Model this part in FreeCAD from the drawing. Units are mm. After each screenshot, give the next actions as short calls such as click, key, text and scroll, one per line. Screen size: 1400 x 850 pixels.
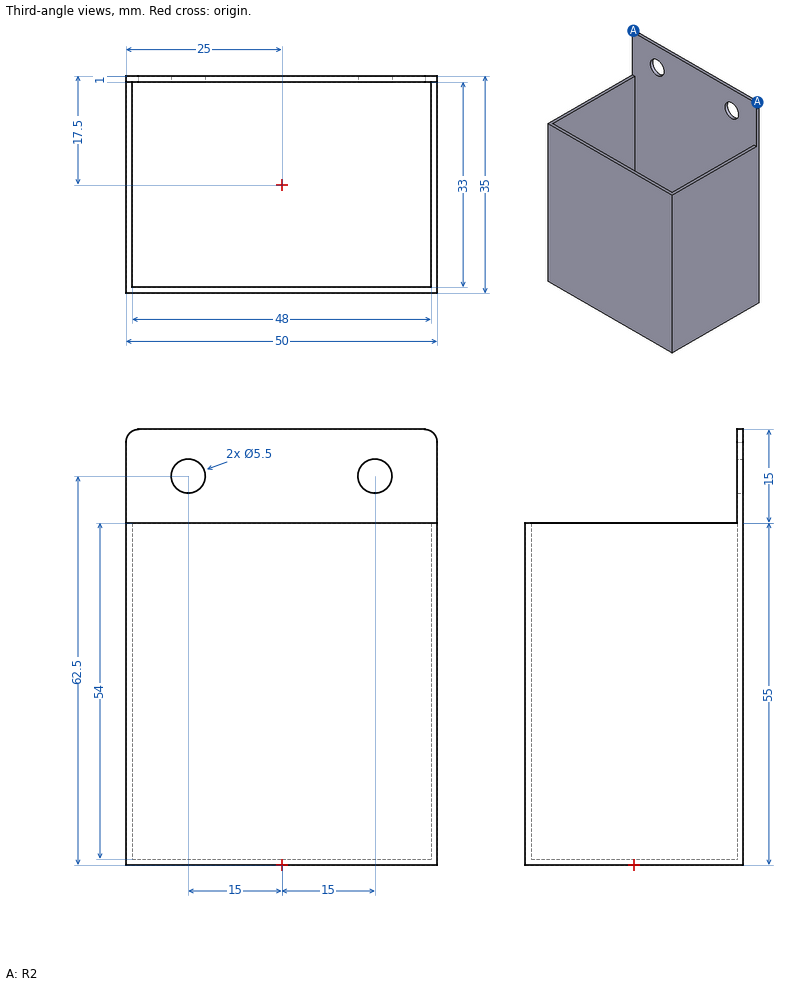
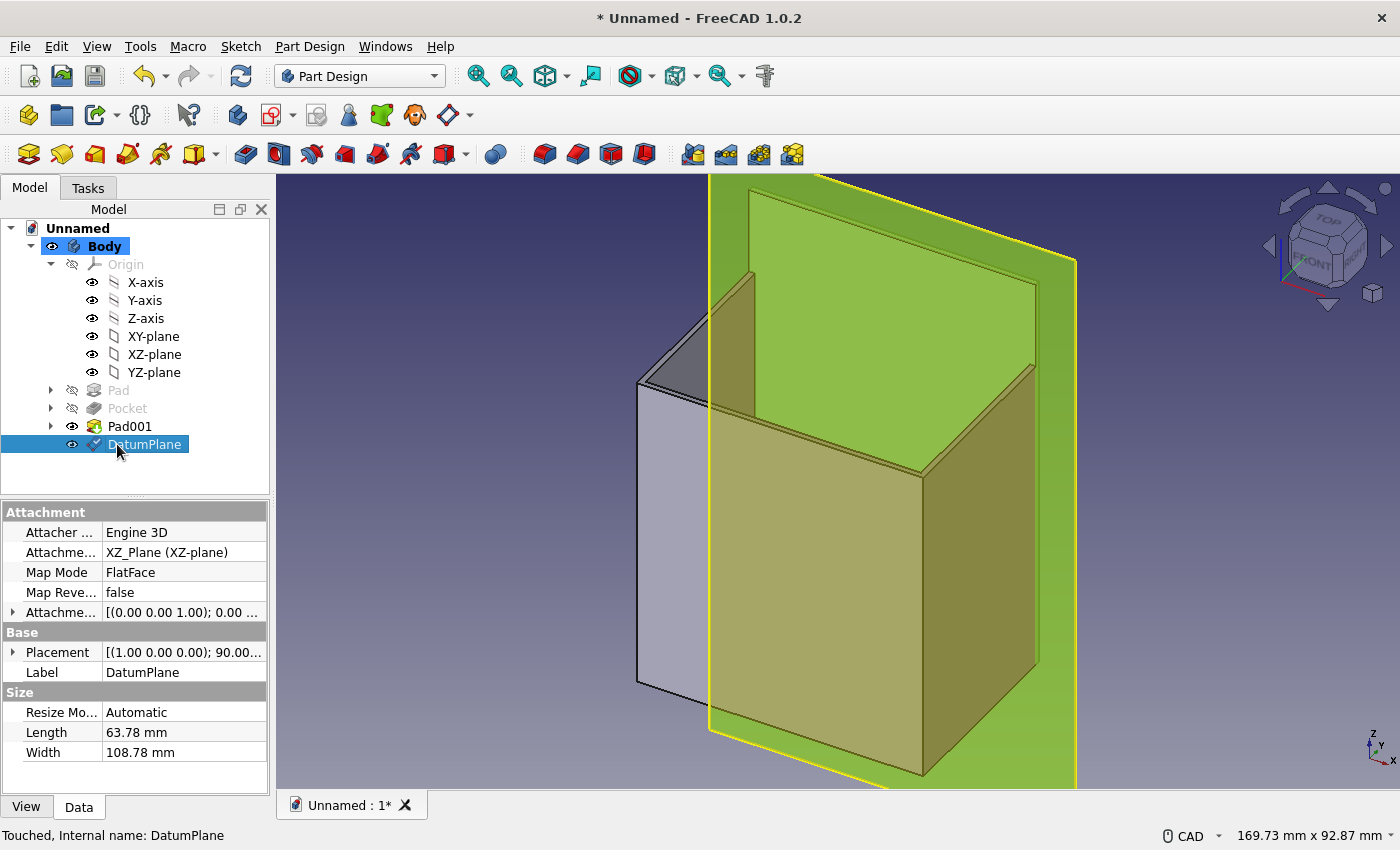
click(270, 116)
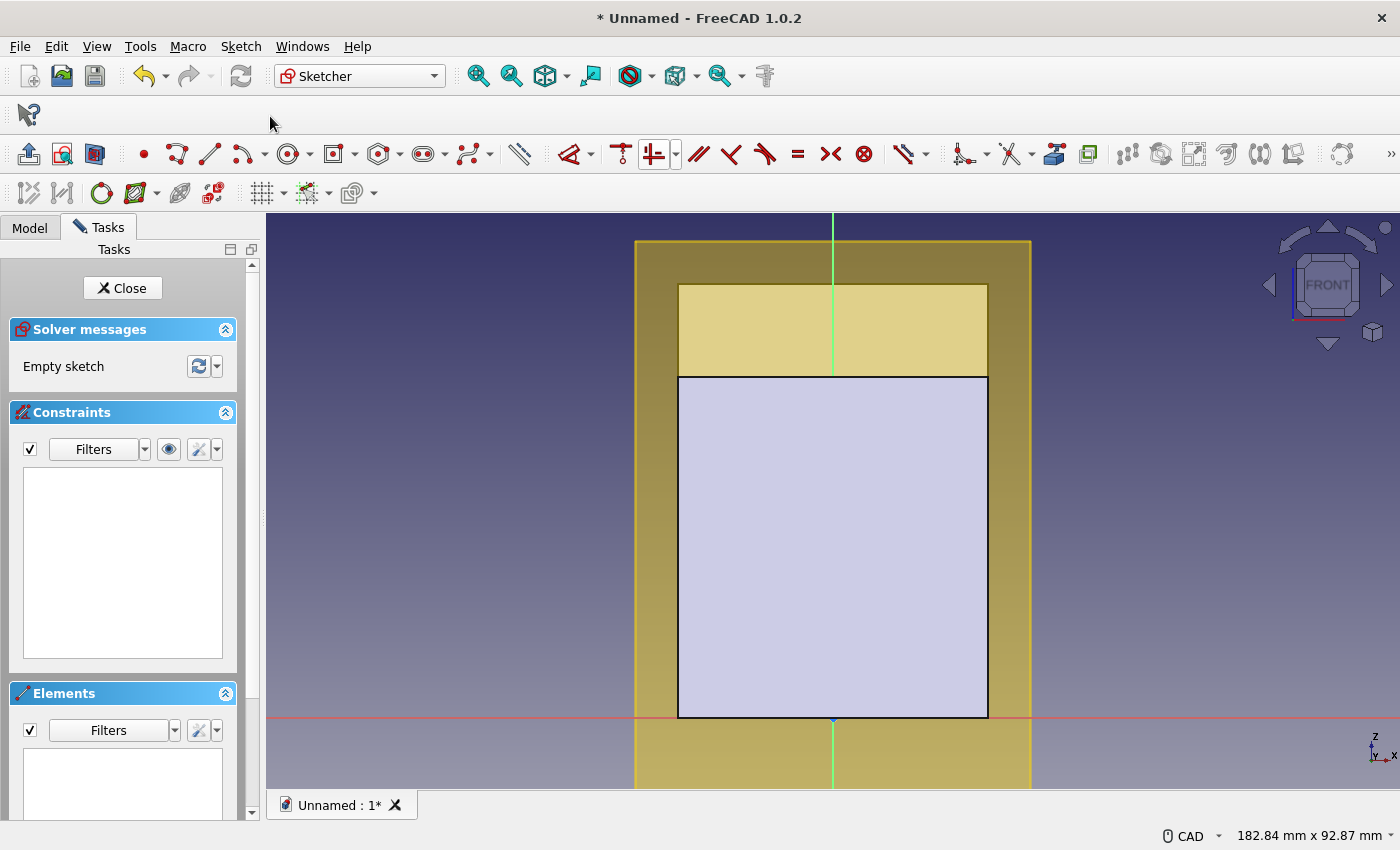
key(q)
key(s)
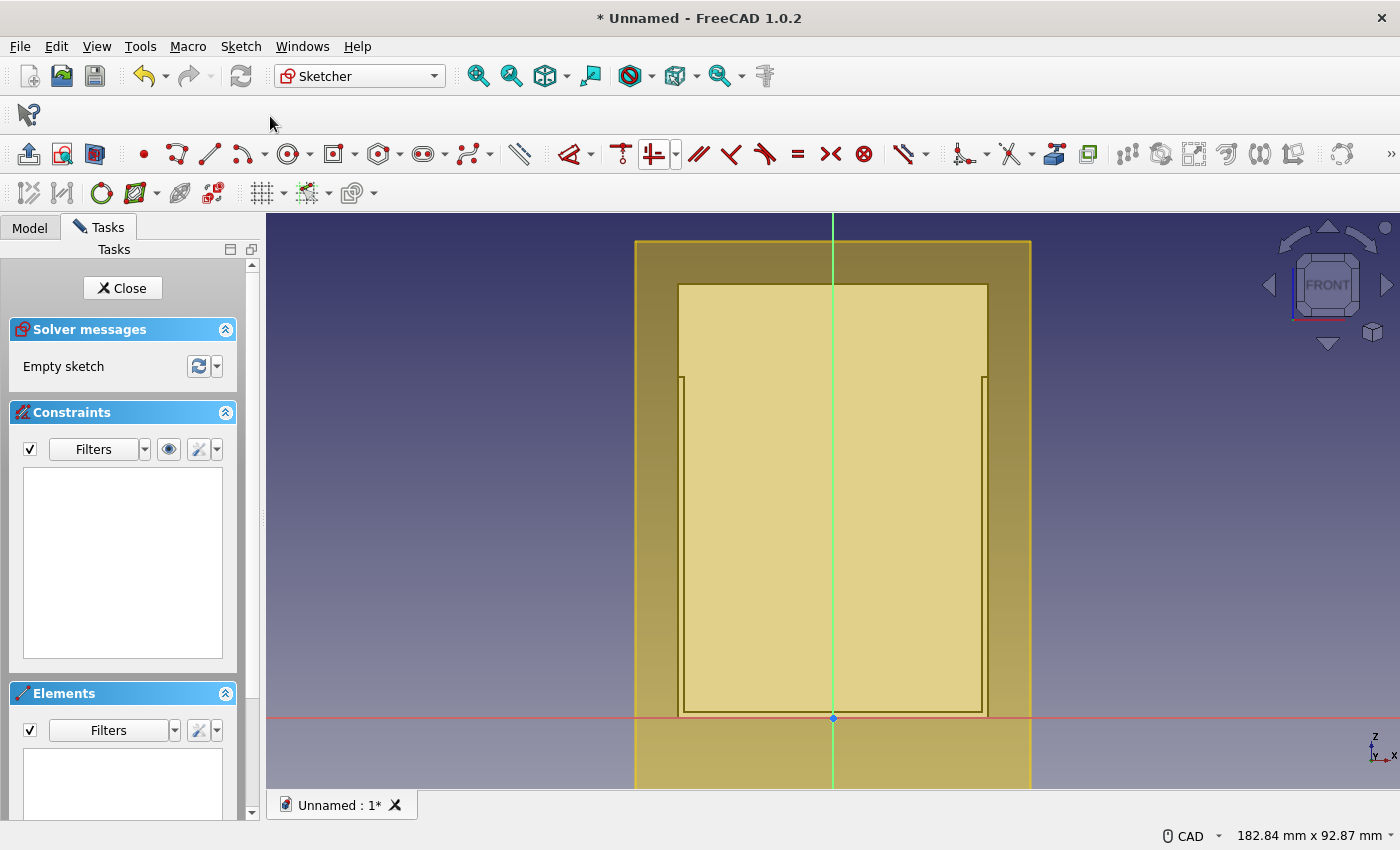
click(288, 154)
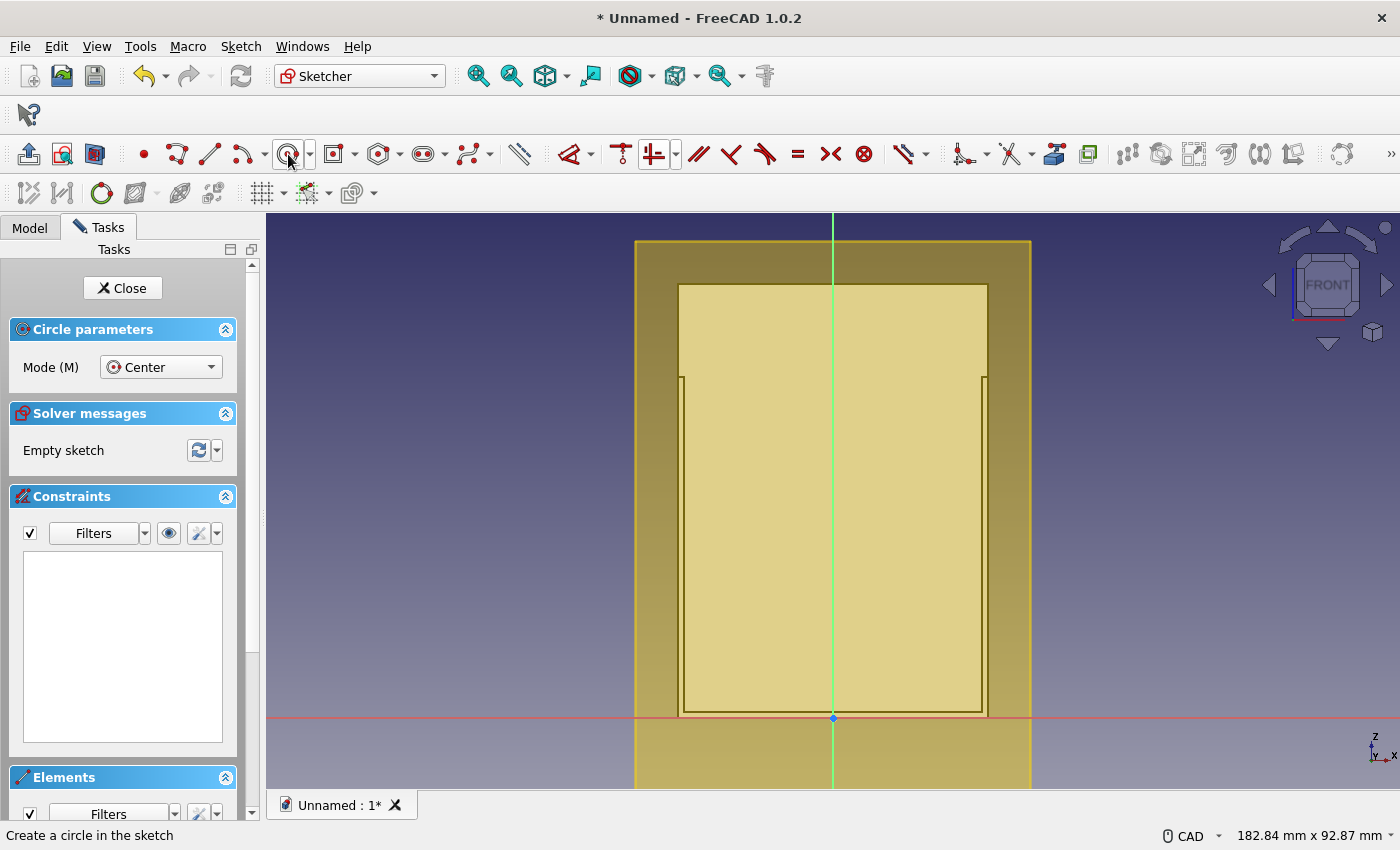
scroll(740, 330, up, 2)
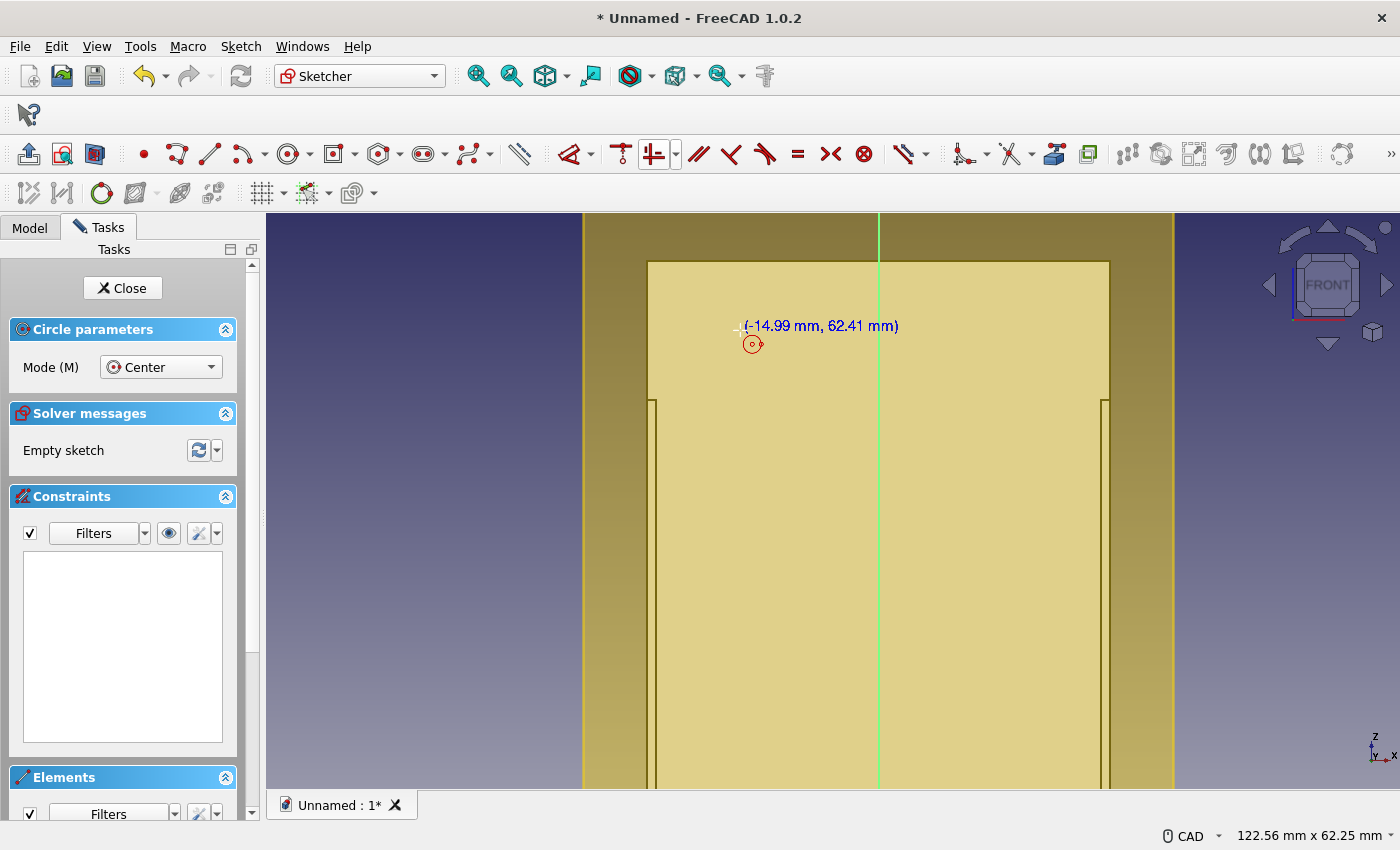
click(740, 331)
click(758, 313)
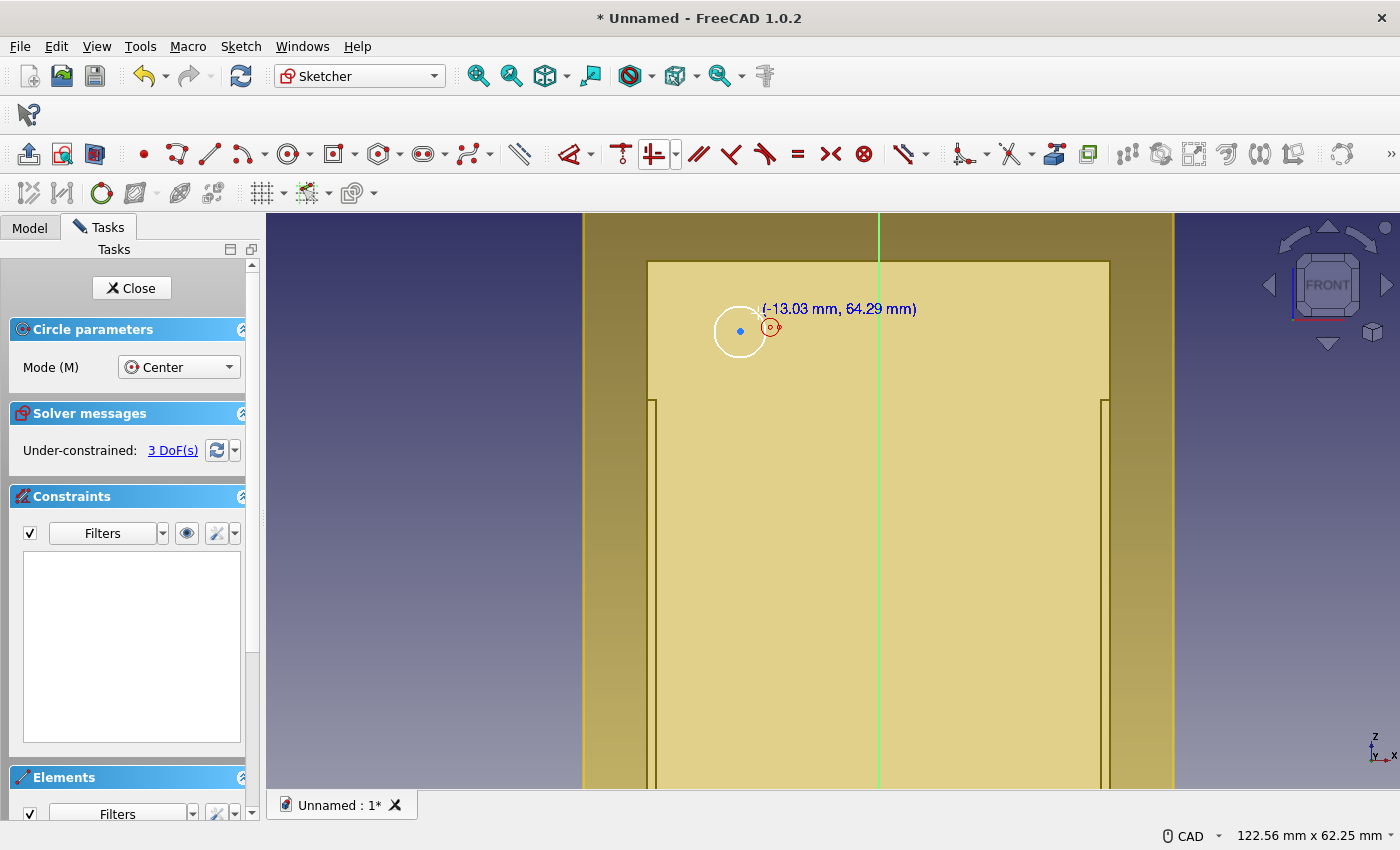
click(1017, 331)
click(1035, 313)
key(Escape)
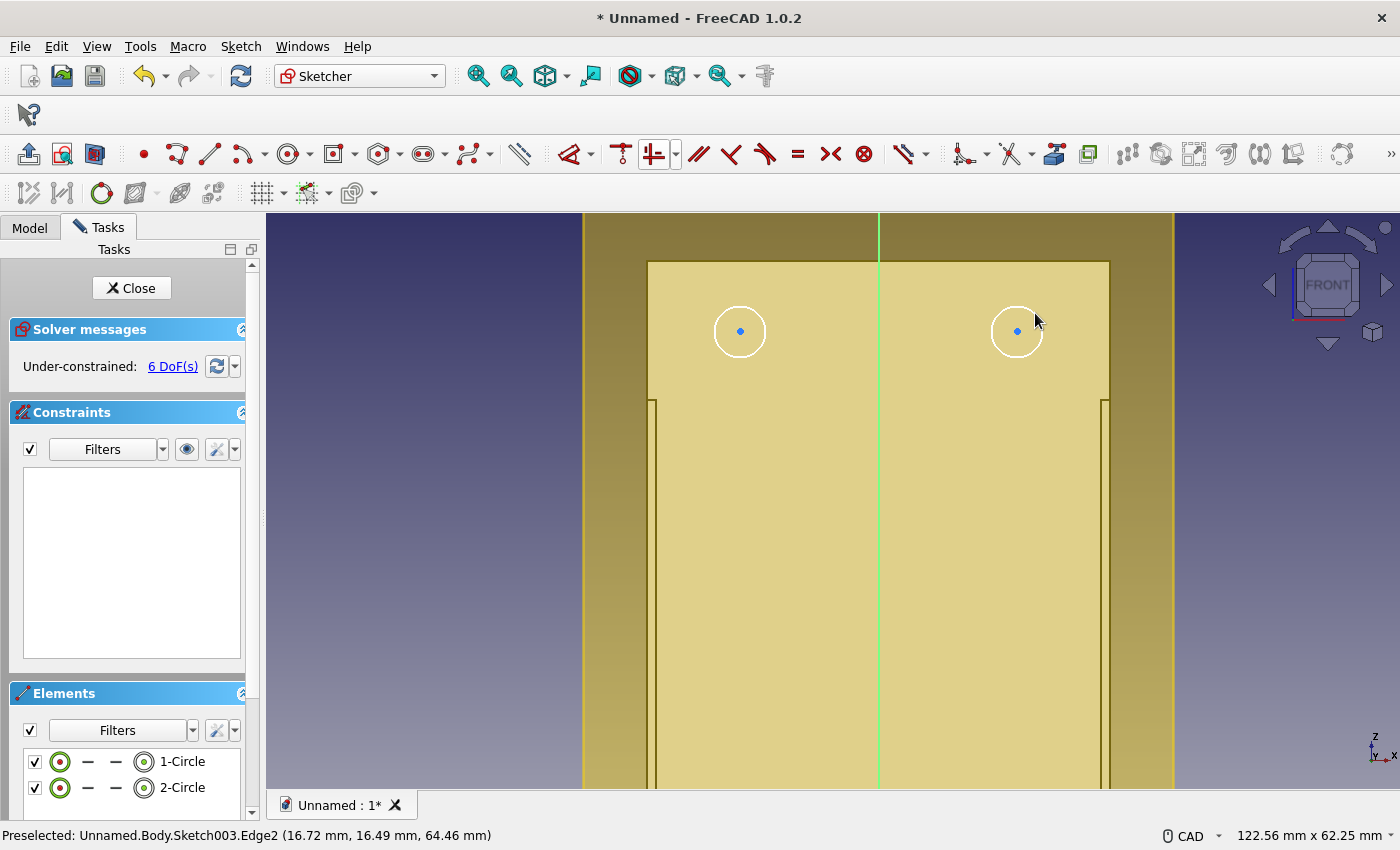
click(758, 314)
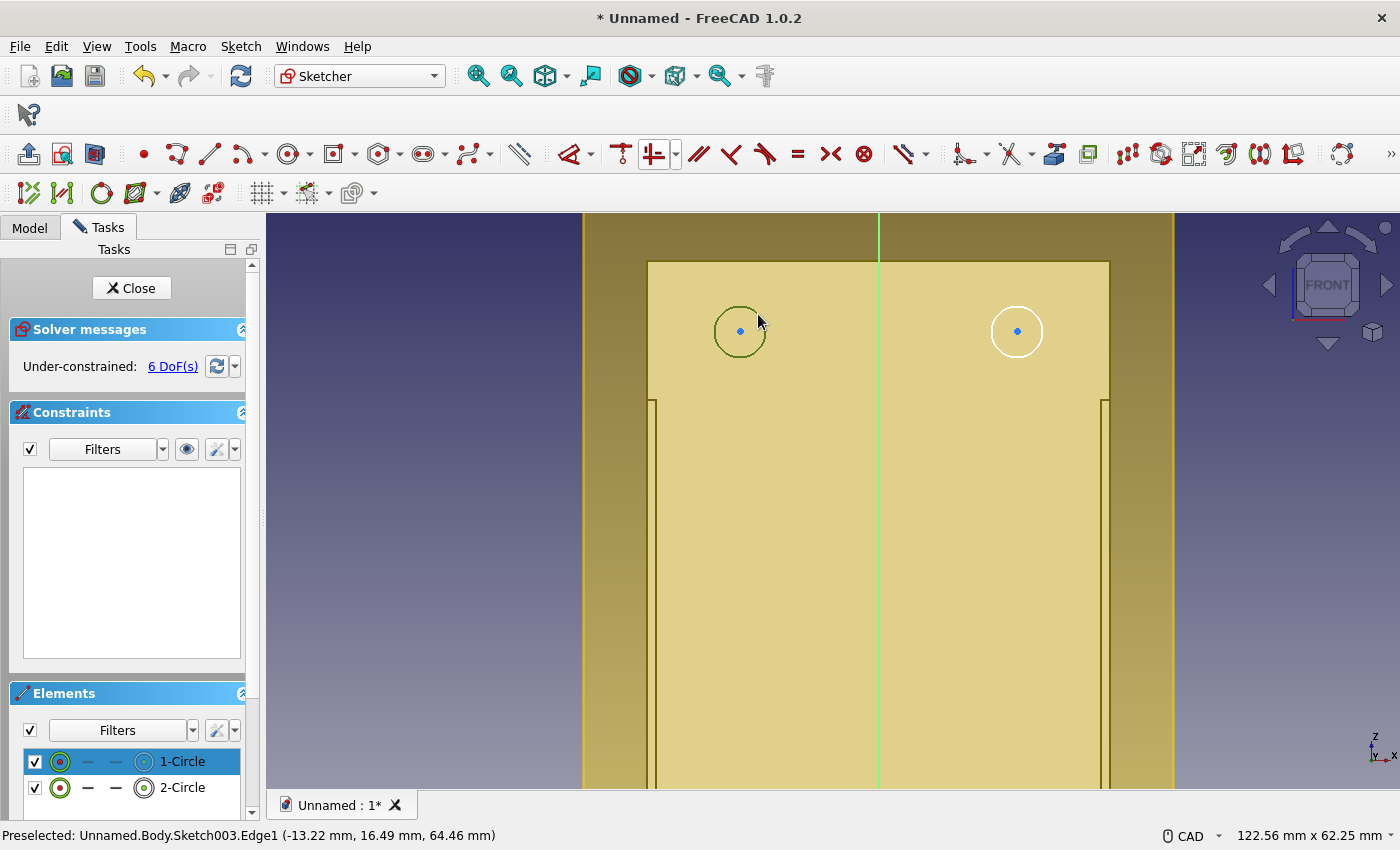
click(1035, 314)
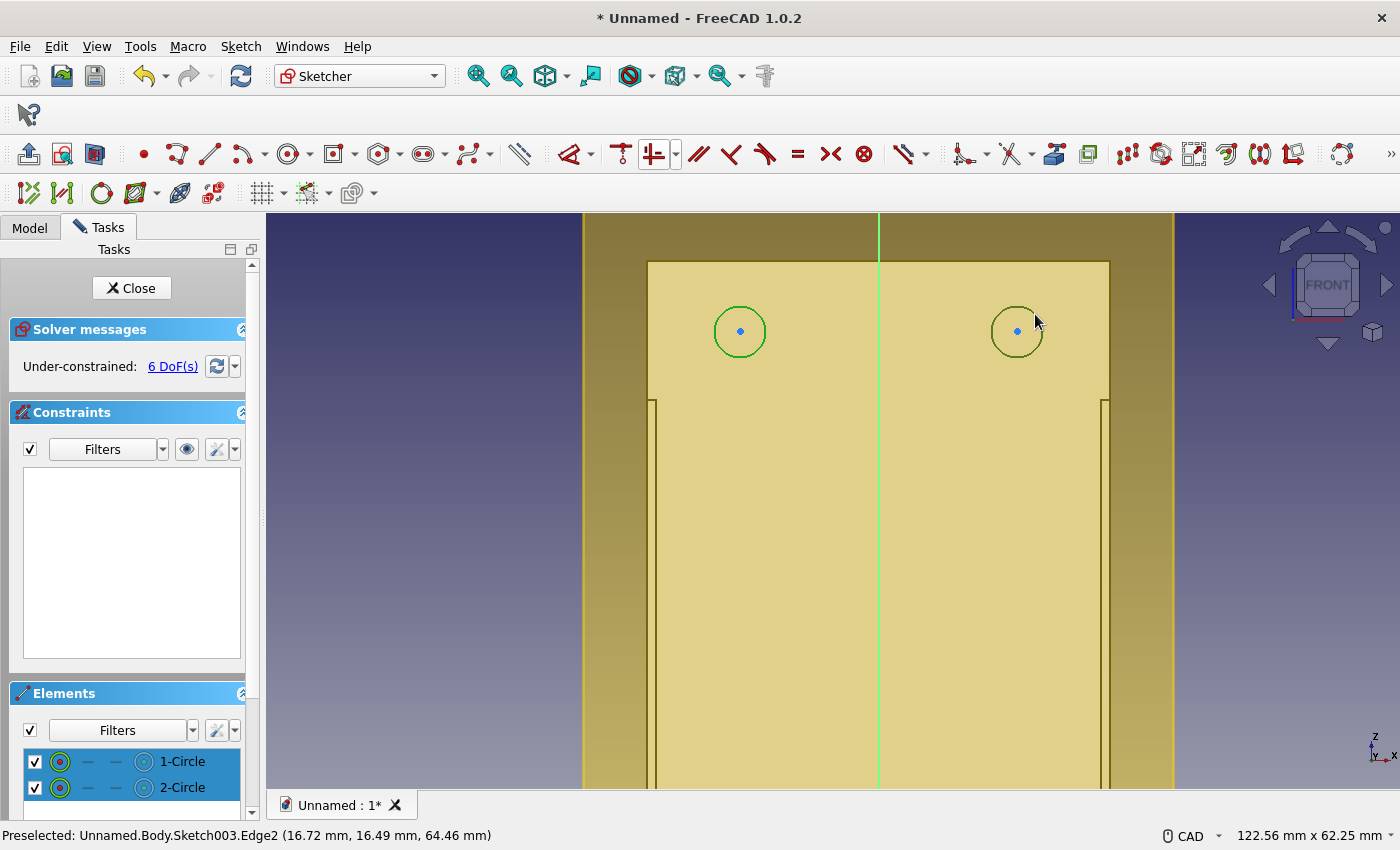
key(e)